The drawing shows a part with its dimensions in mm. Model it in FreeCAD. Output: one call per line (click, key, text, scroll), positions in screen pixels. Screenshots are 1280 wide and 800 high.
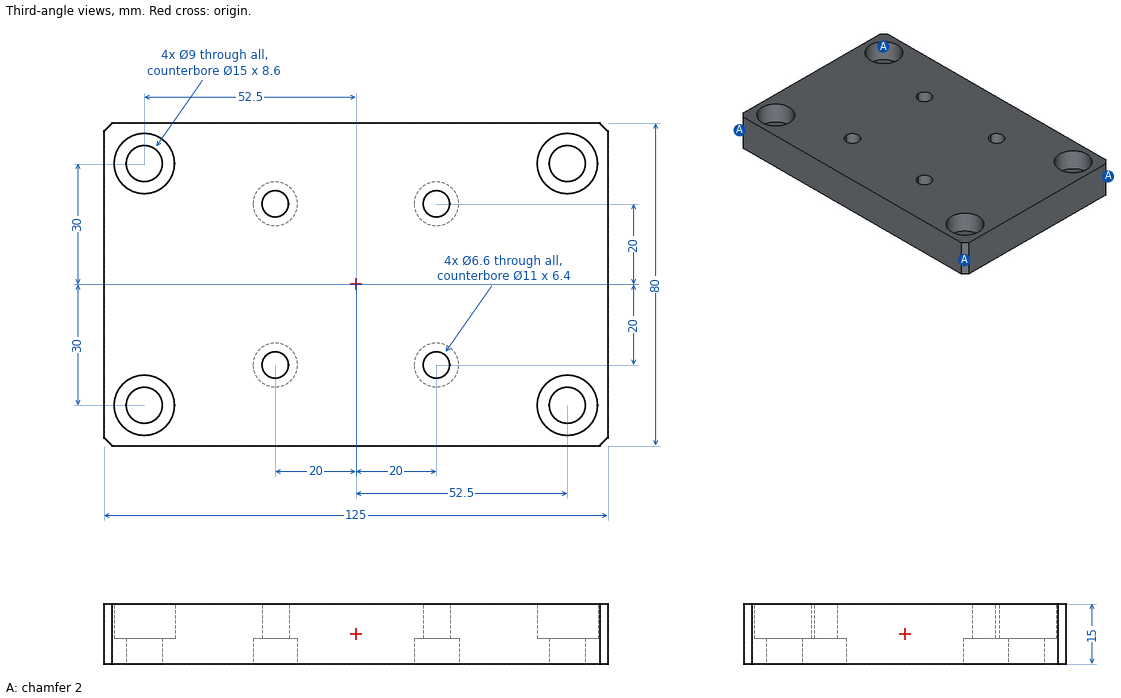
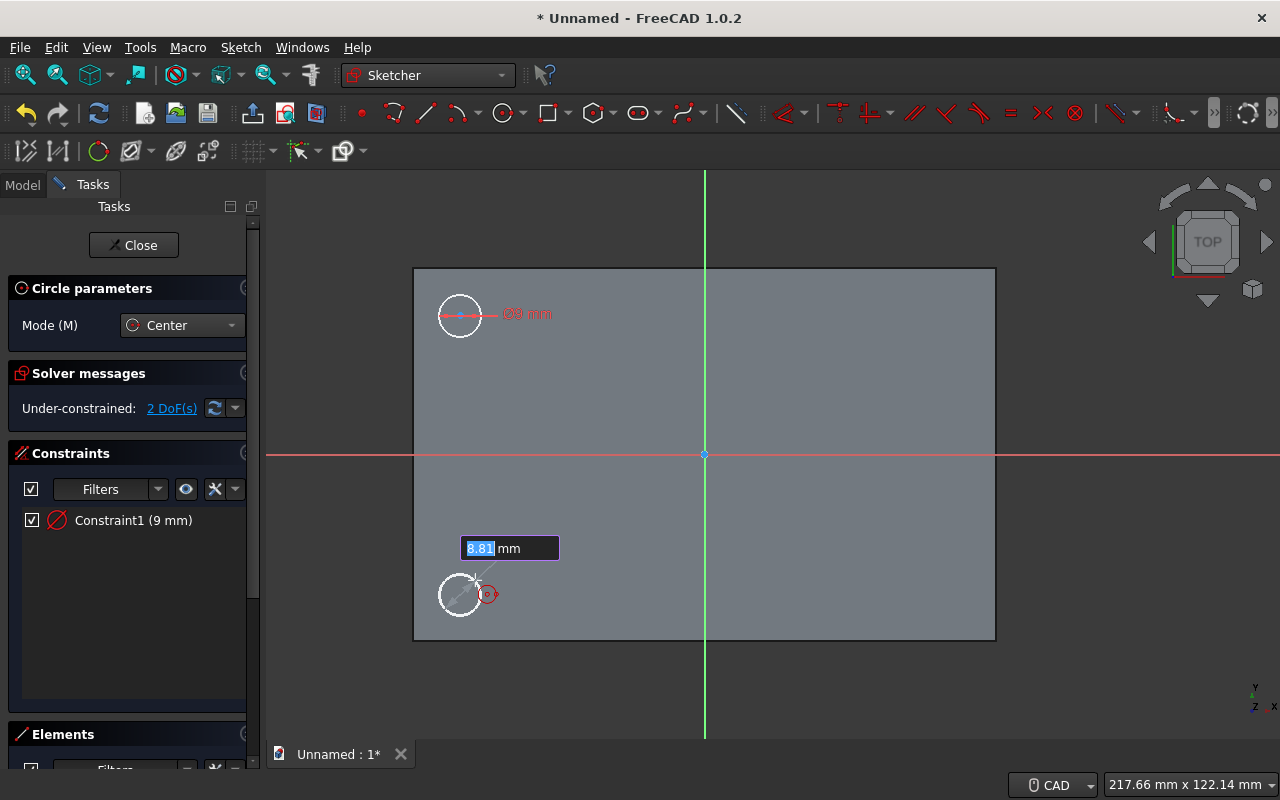
text(9)
key(Return)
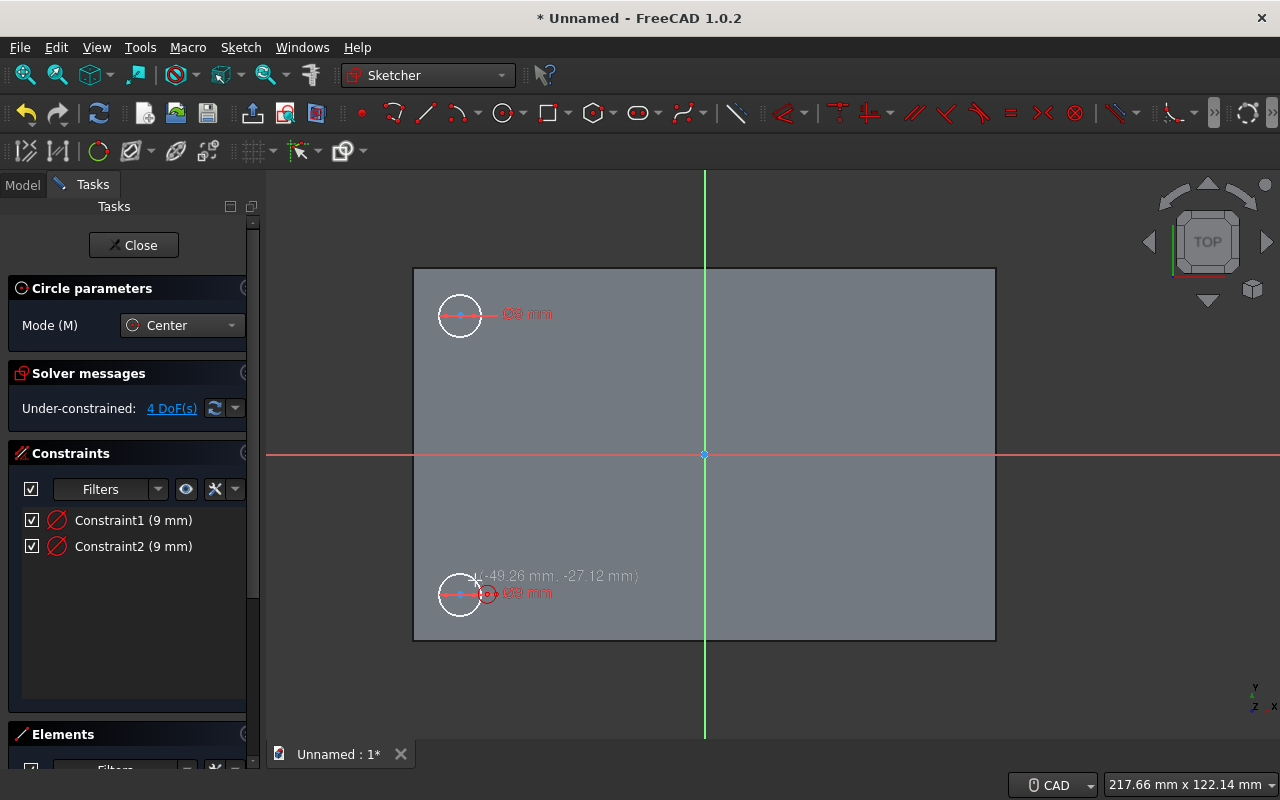
click(949, 594)
move(964, 580)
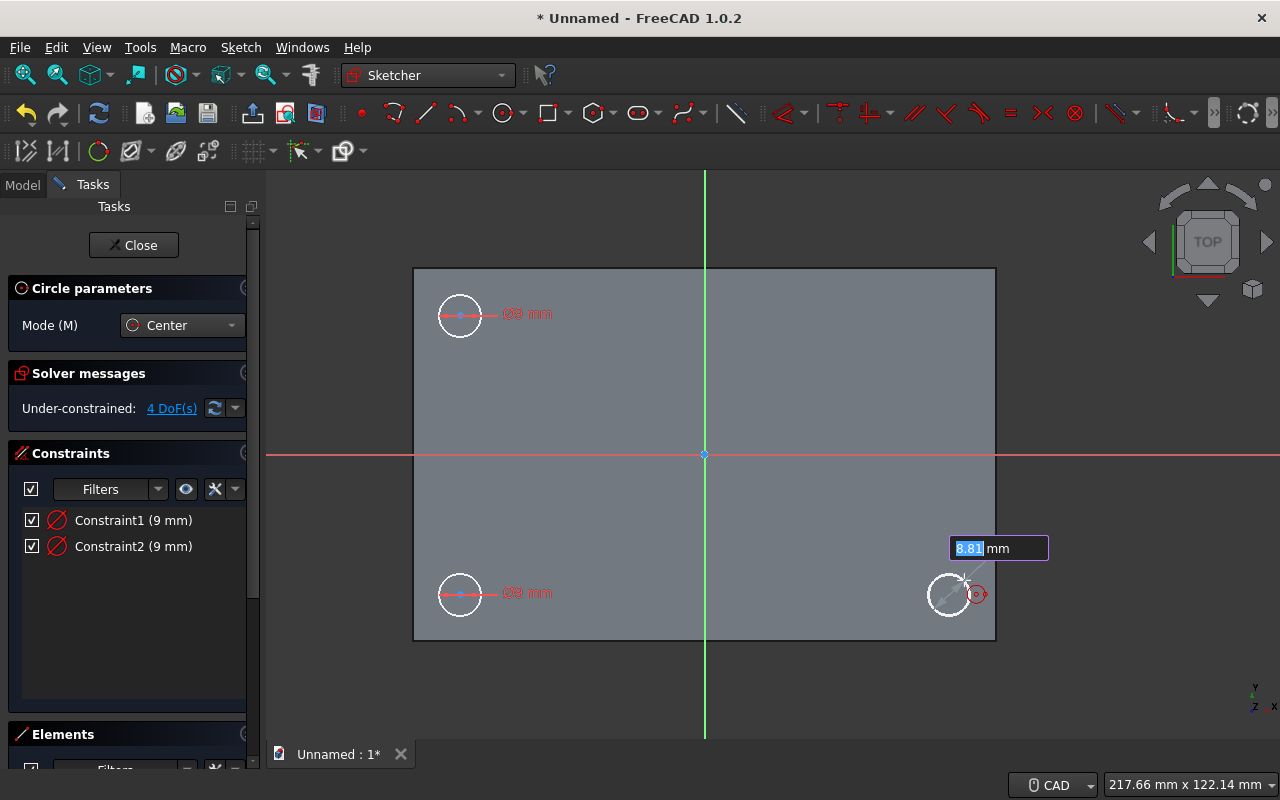
text(9)
key(Return)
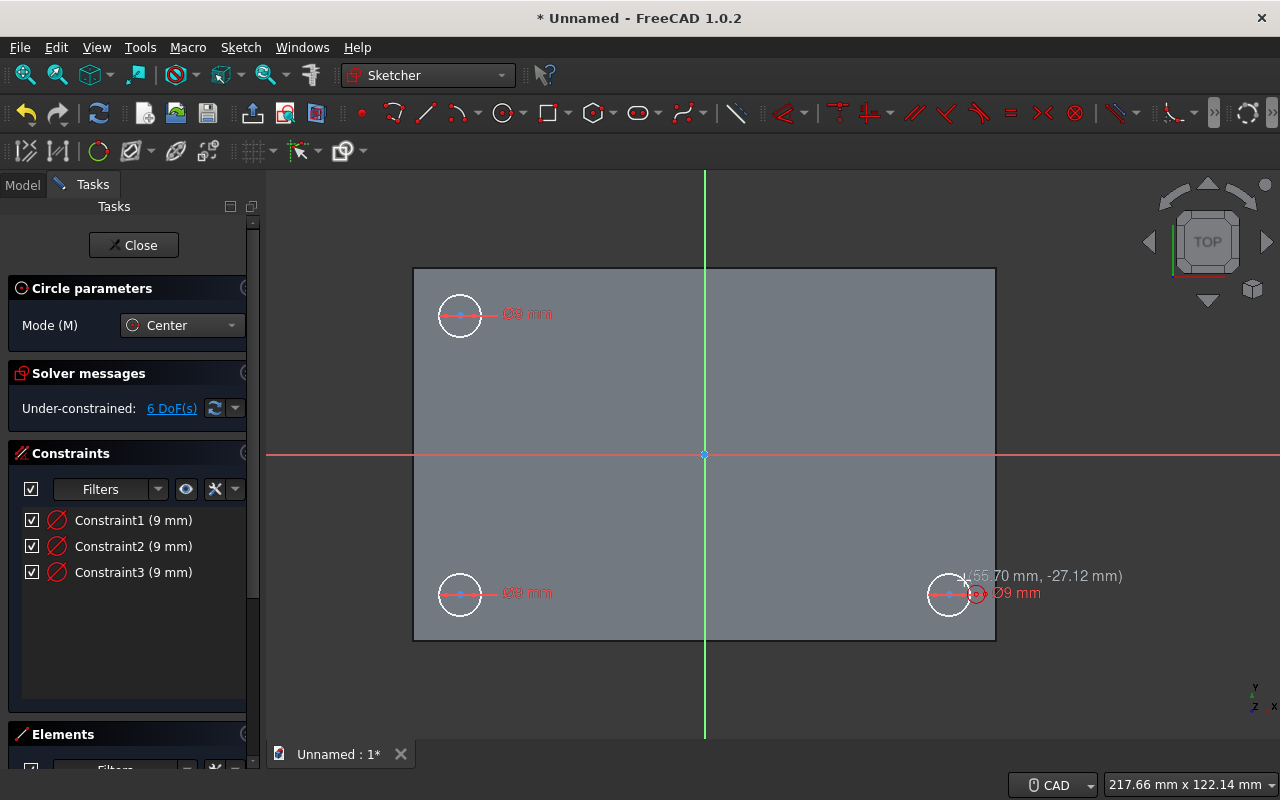
click(949, 315)
move(964, 300)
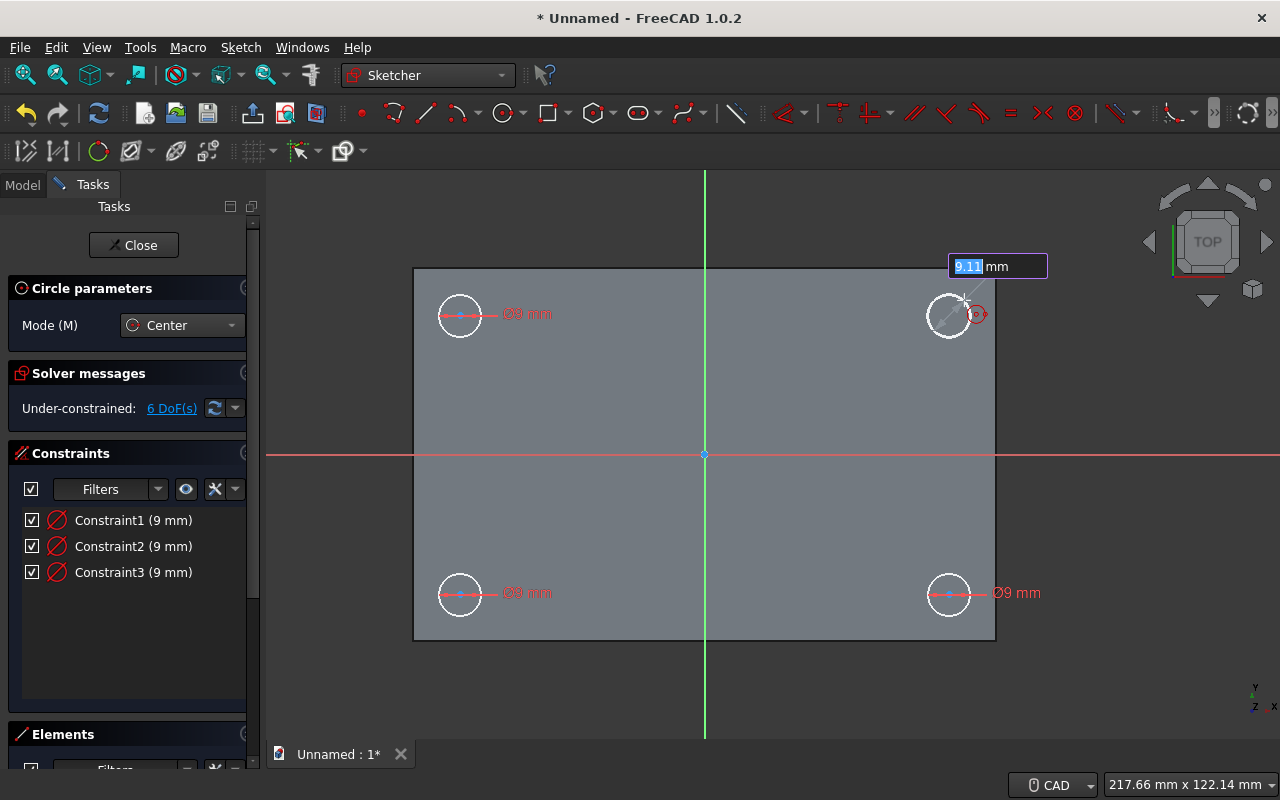
text(9)
key(Return)
key(Escape)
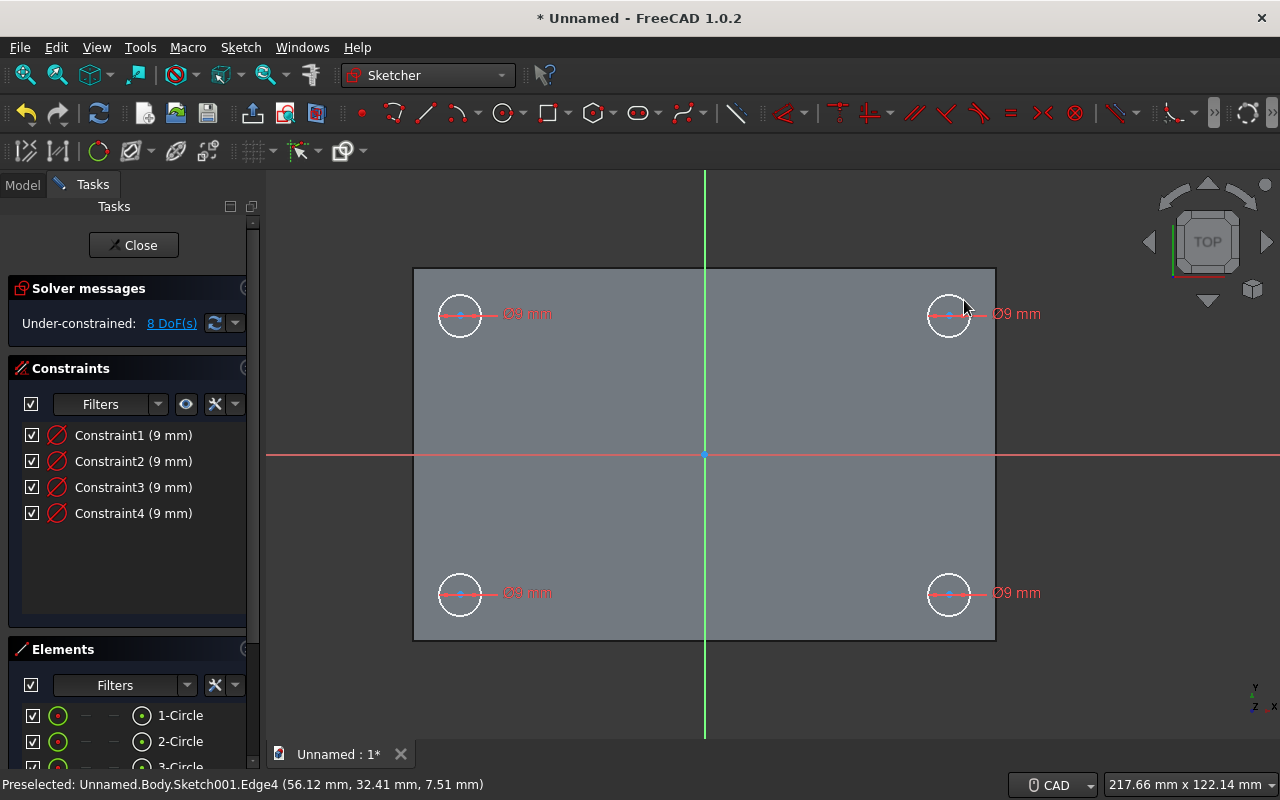
click(460, 316)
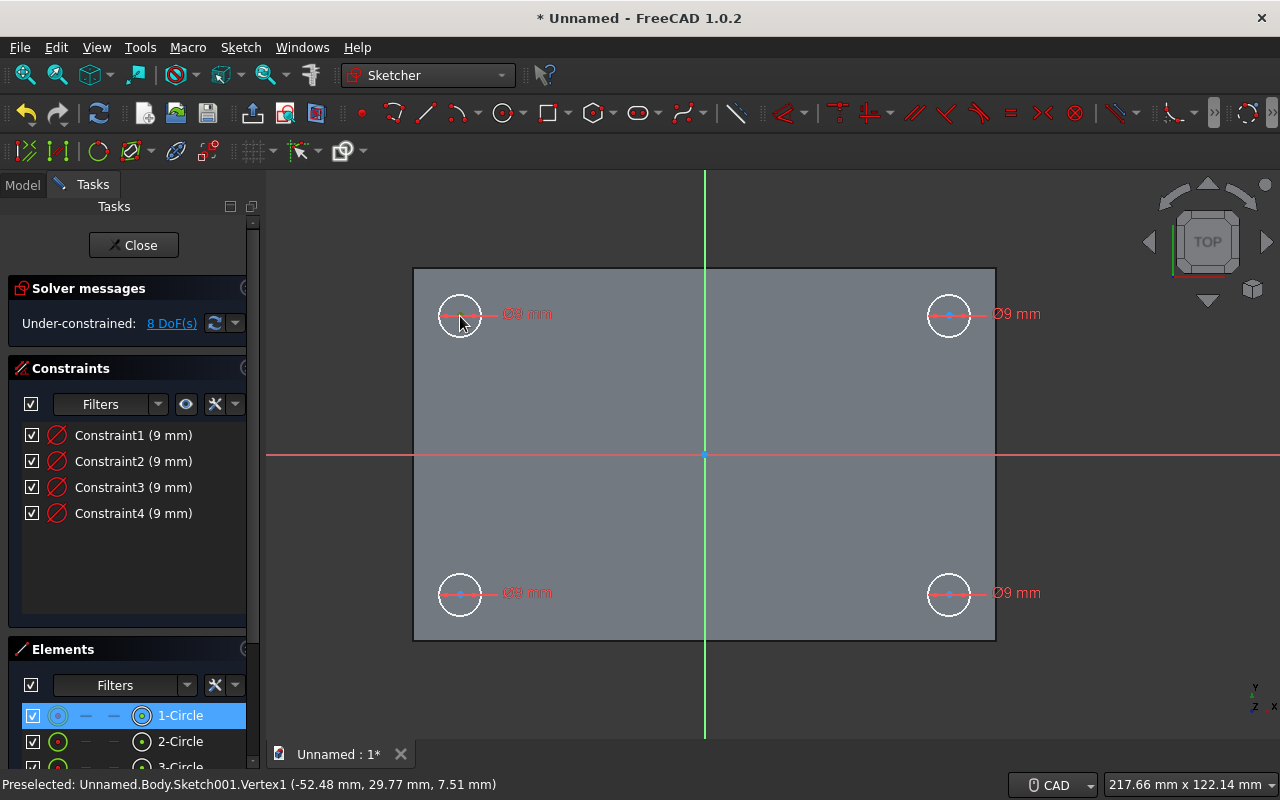
click(460, 595)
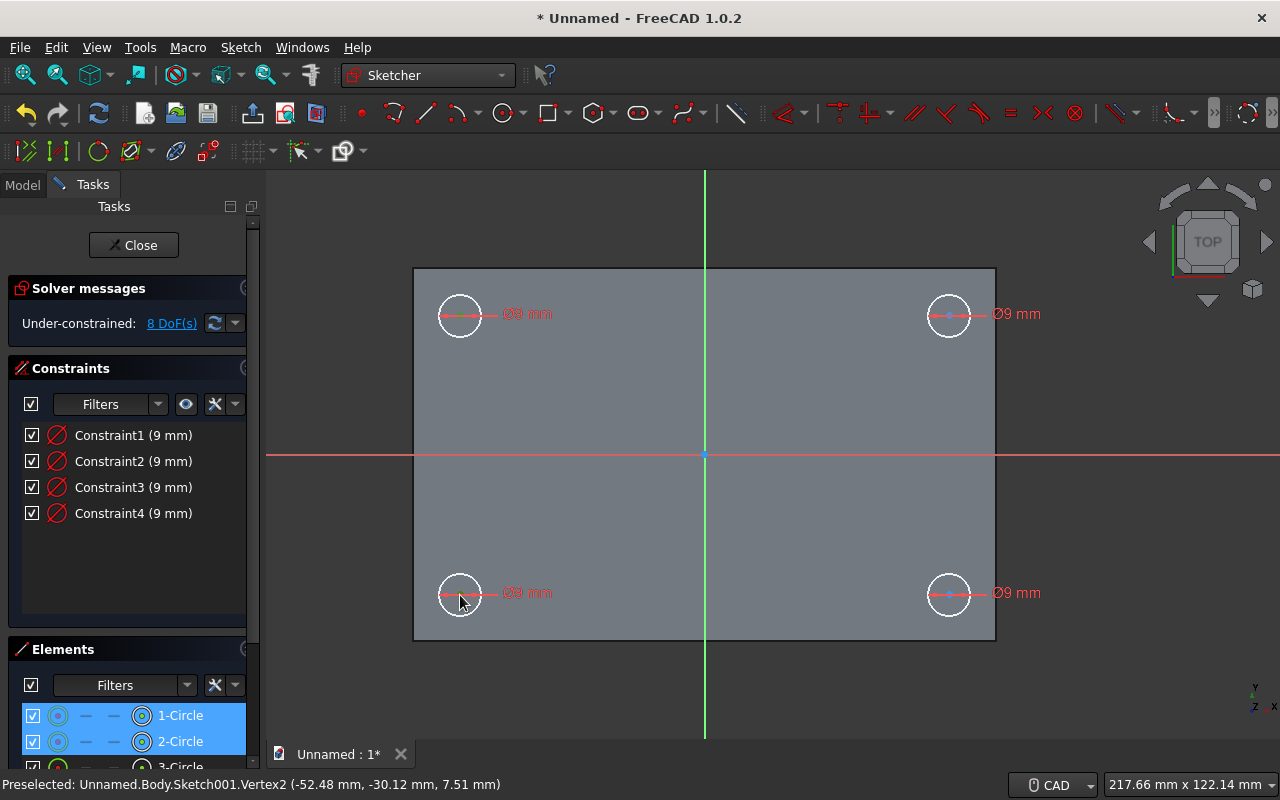
key(v)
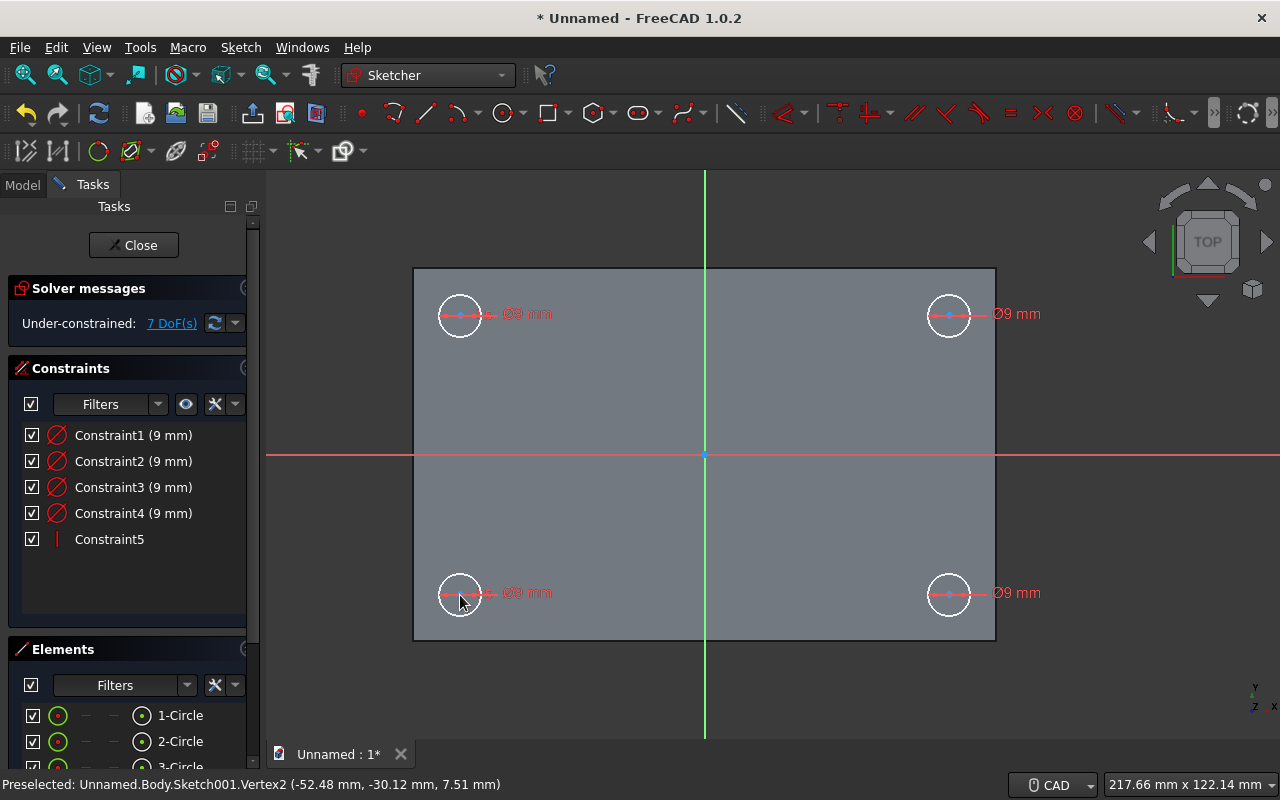
click(460, 595)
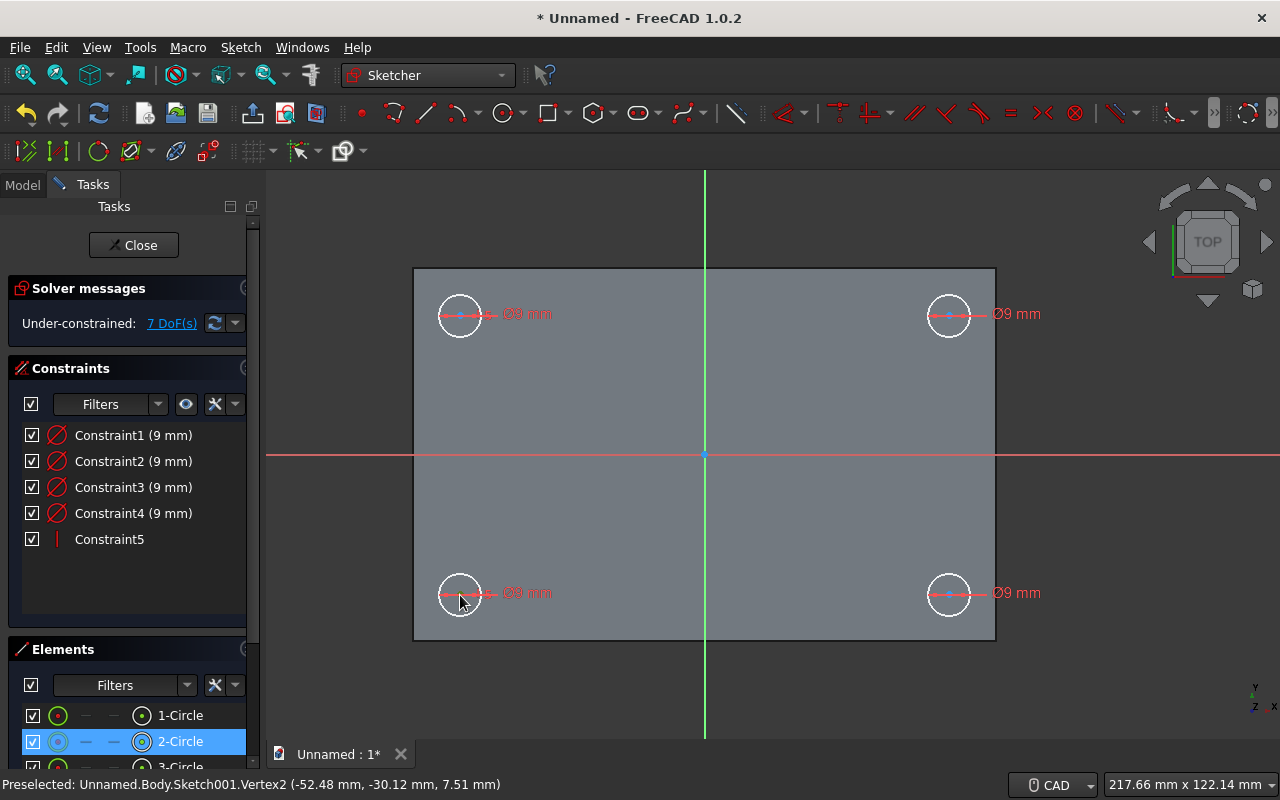
click(949, 595)